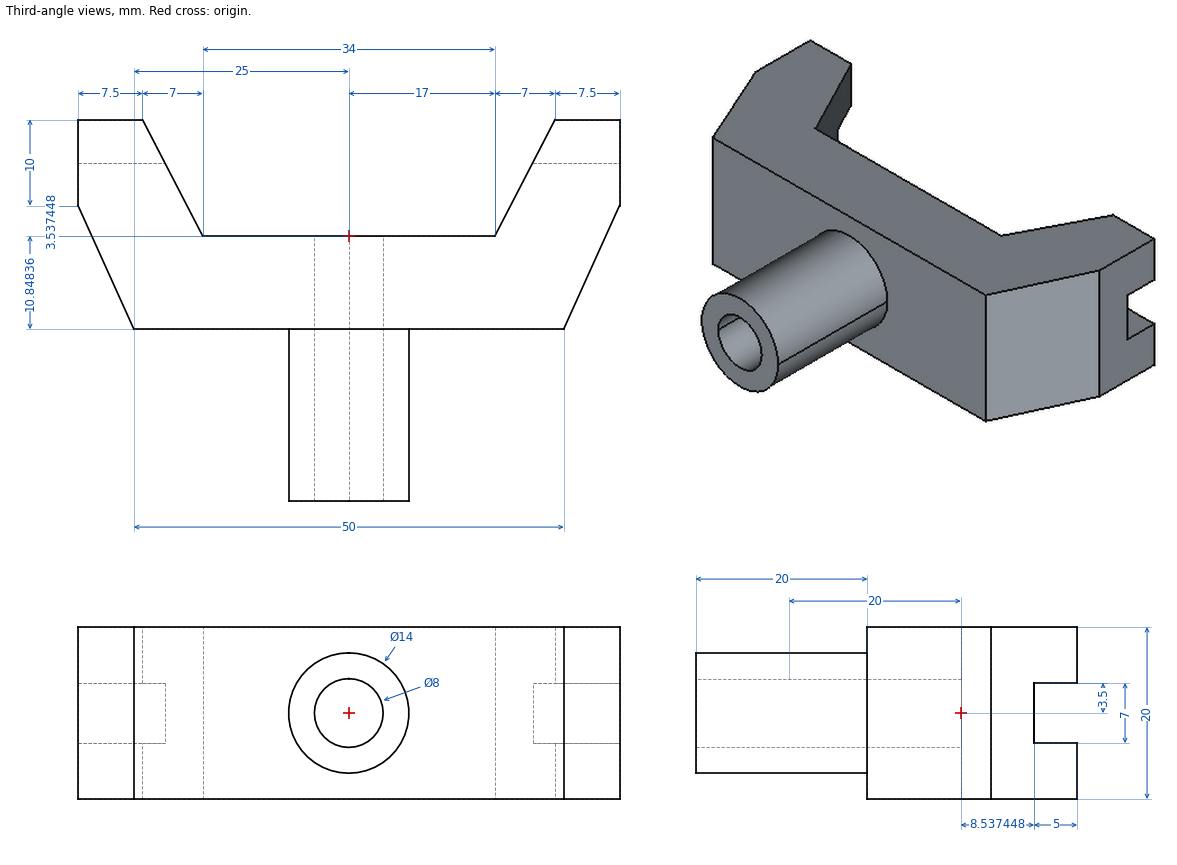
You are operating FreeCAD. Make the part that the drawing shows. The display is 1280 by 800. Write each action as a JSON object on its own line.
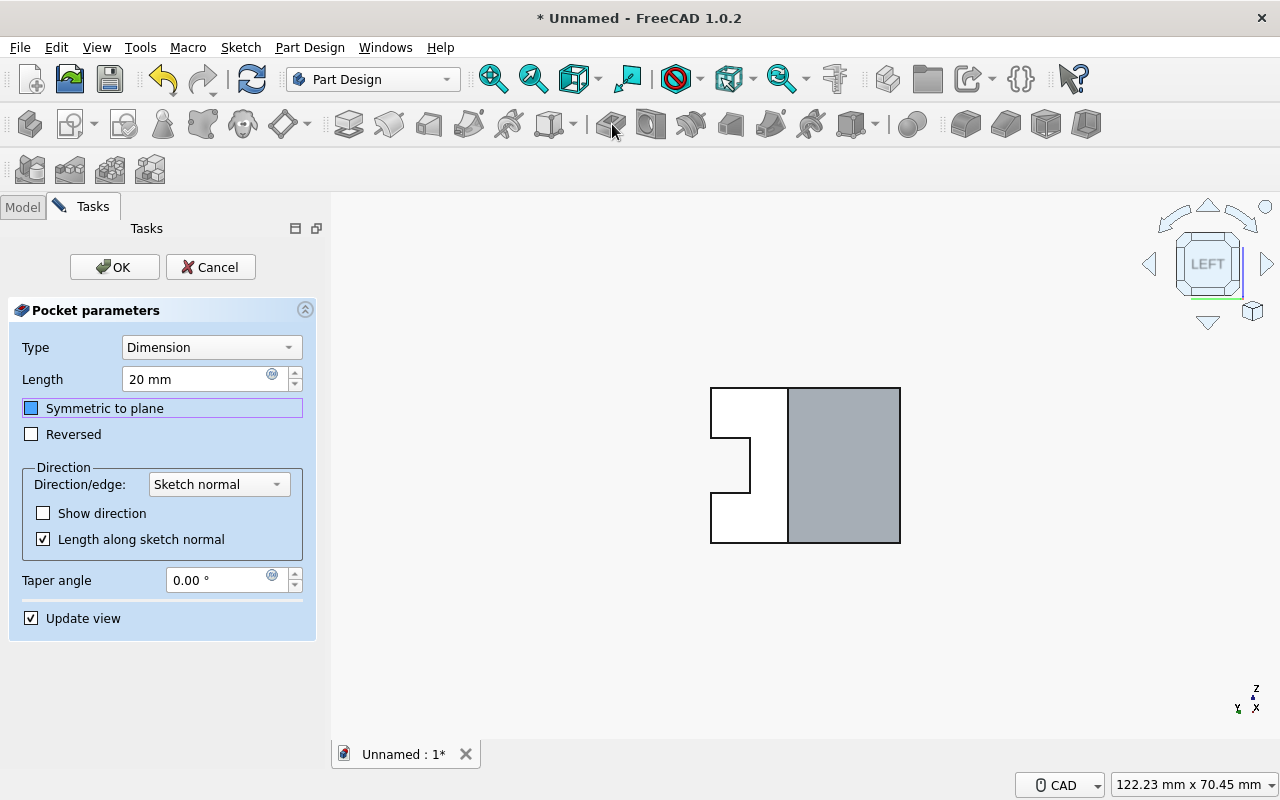
{"action": "left_click", "coordinate": [30, 434]}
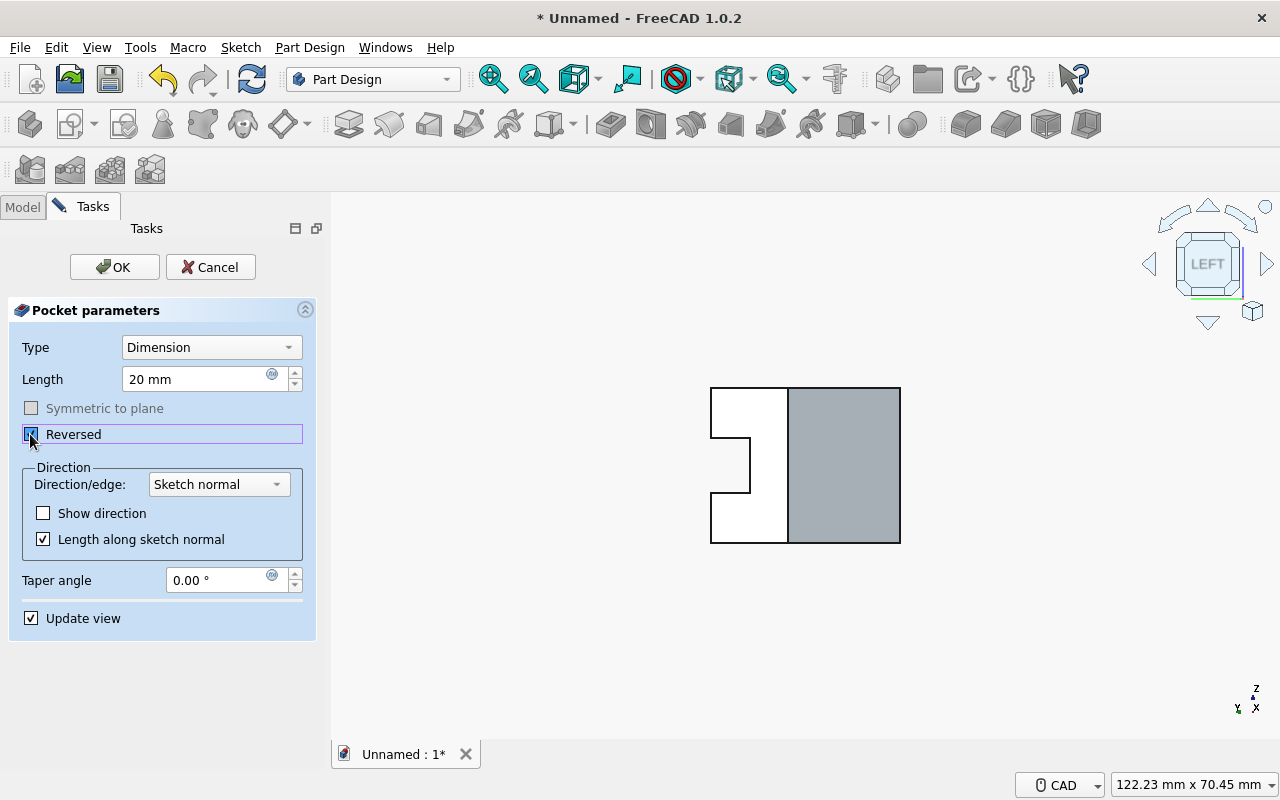
{"action": "left_click", "coordinate": [115, 267]}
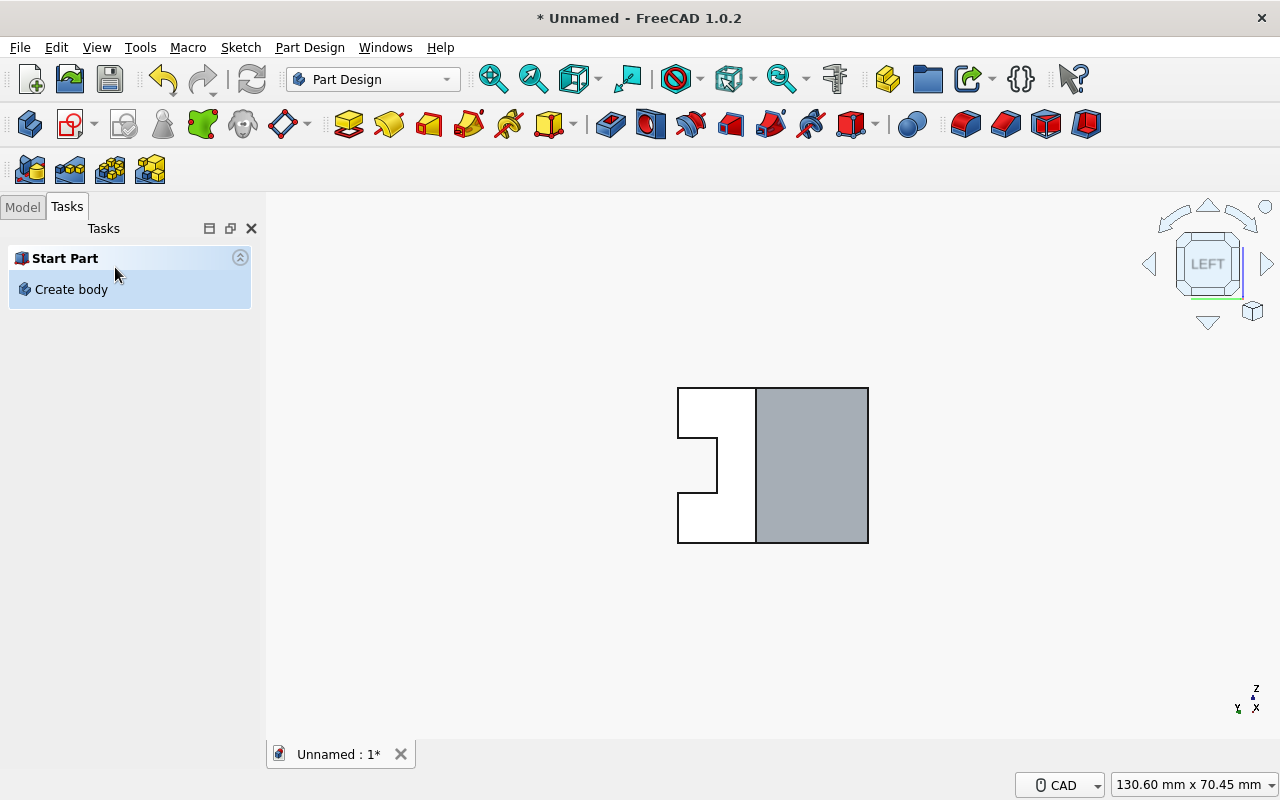
{"action": "left_click", "coordinate": [494, 80]}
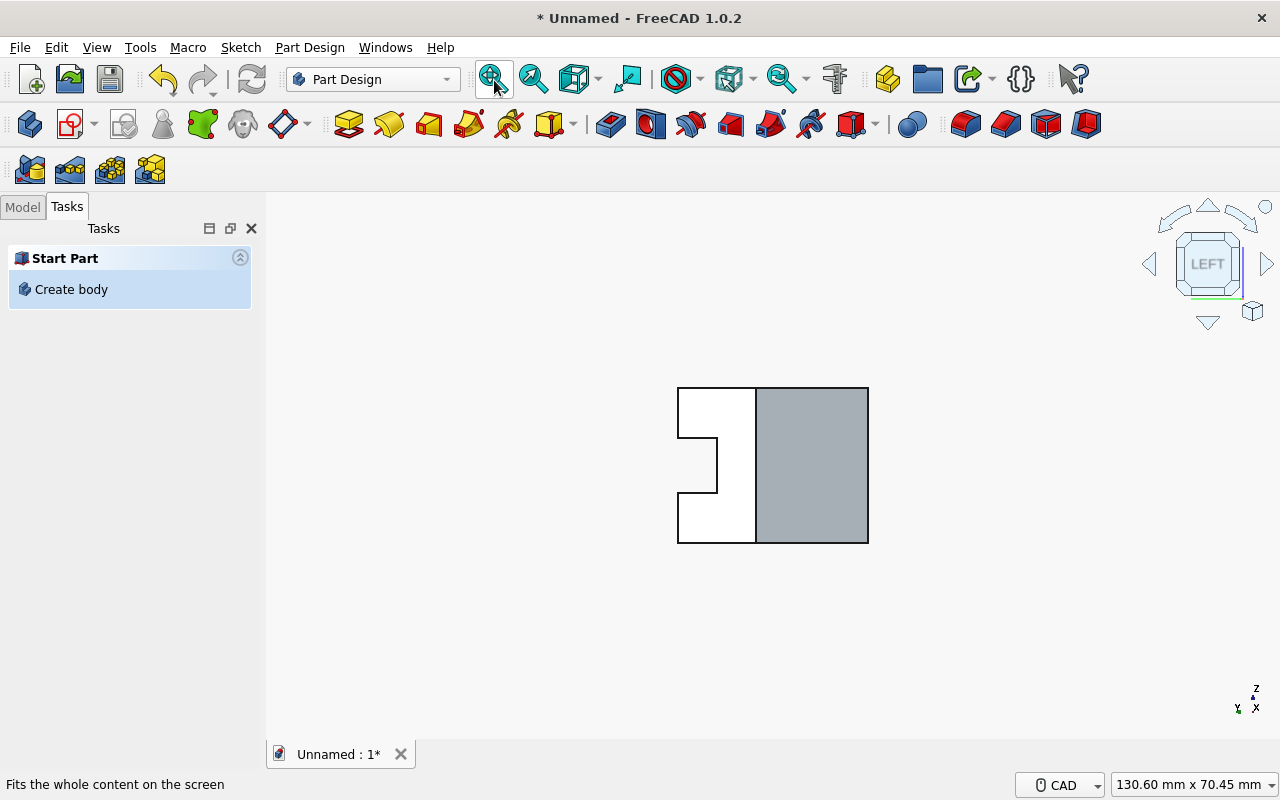
{"action": "key", "text": "0"}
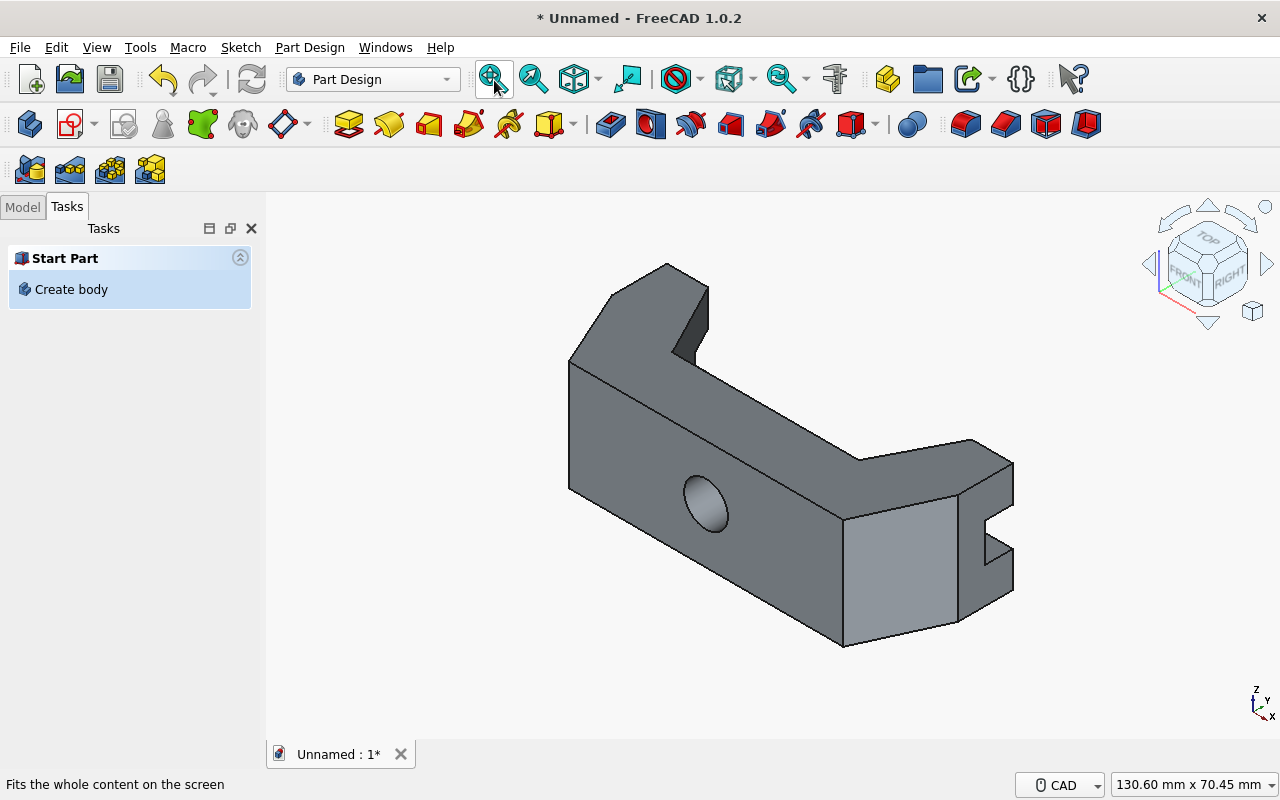
{"action": "left_click", "coordinate": [784, 548]}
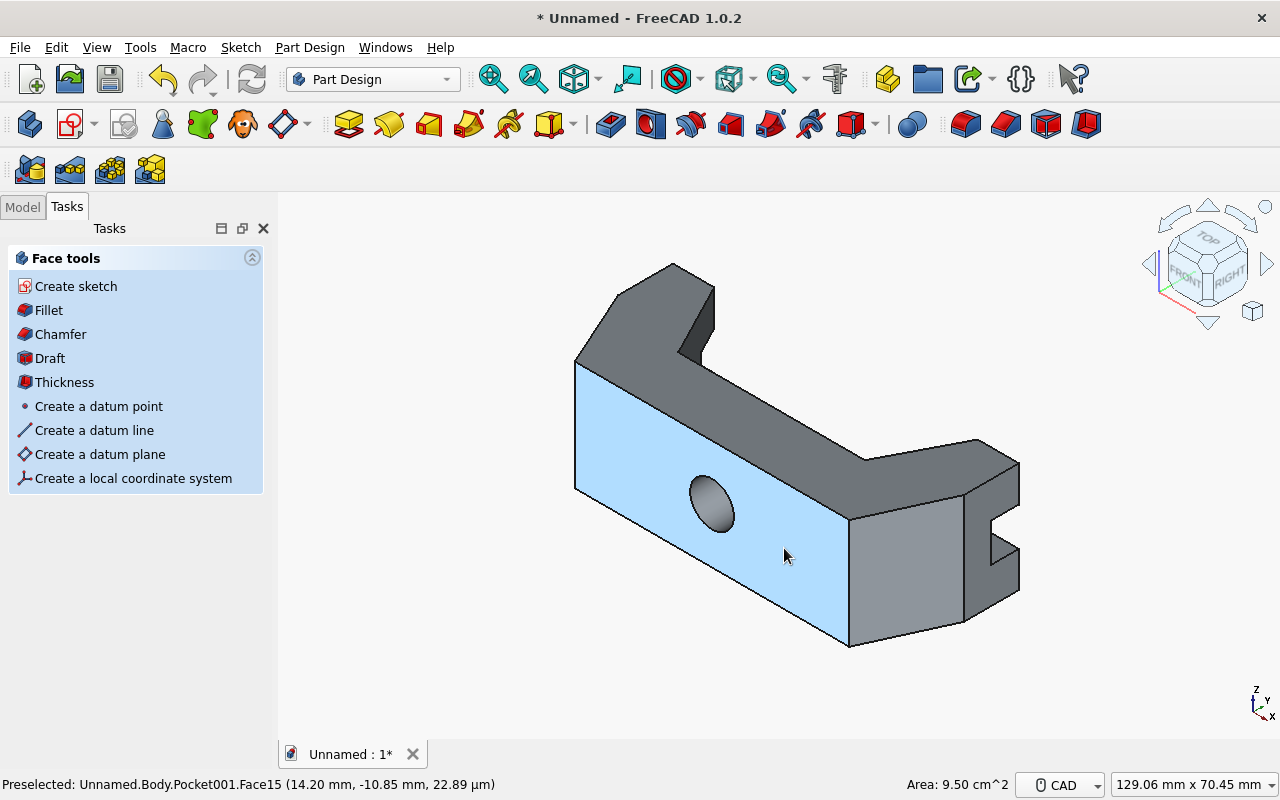
{"action": "left_click", "coordinate": [70, 124]}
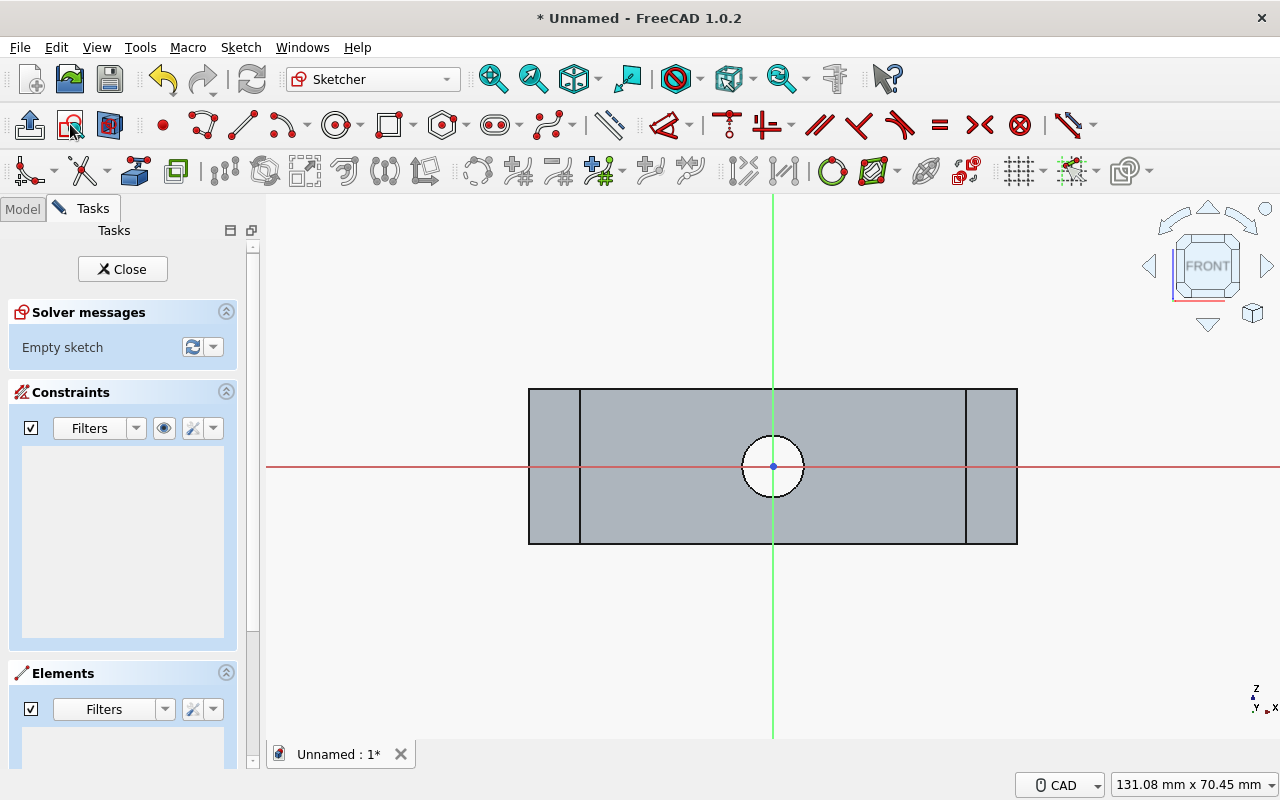
{"action": "scroll", "coordinate": [803, 467], "scroll_direction": "up", "scroll_amount": 6}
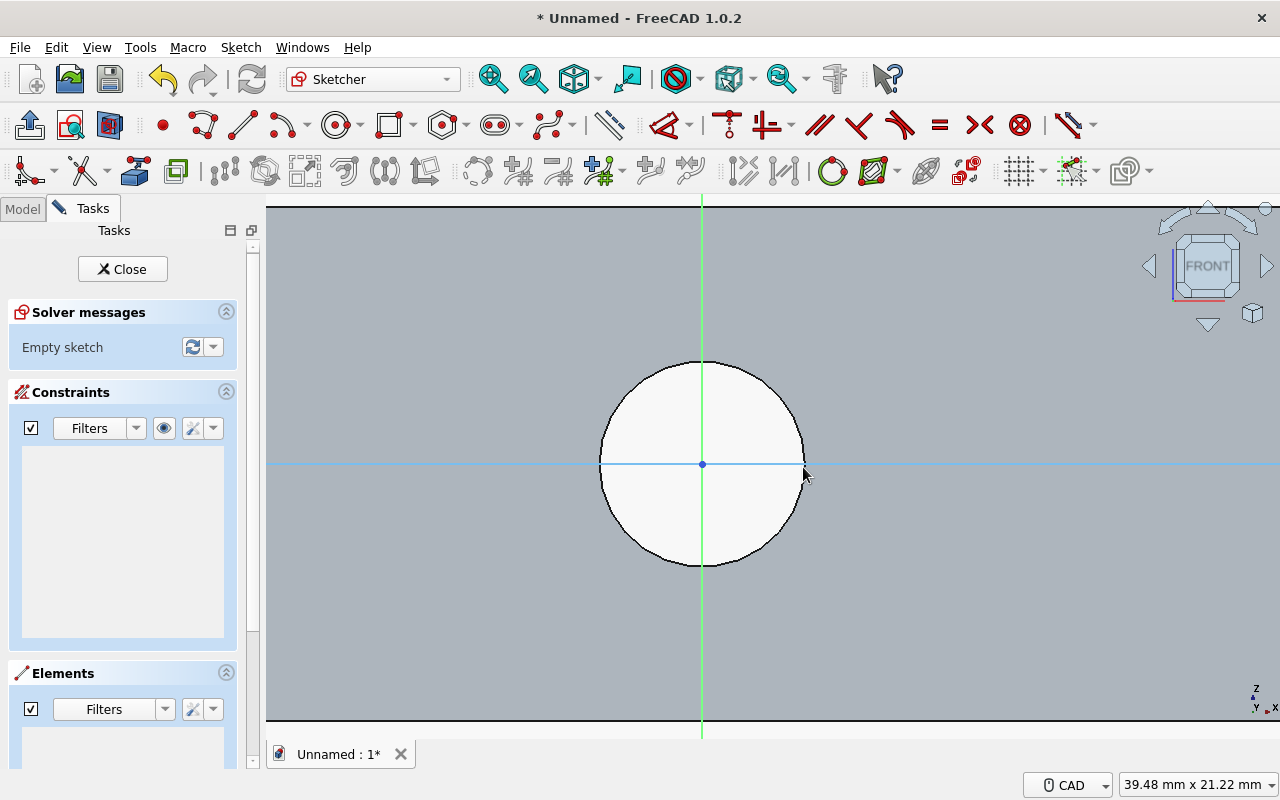
{"action": "left_click", "coordinate": [336, 126]}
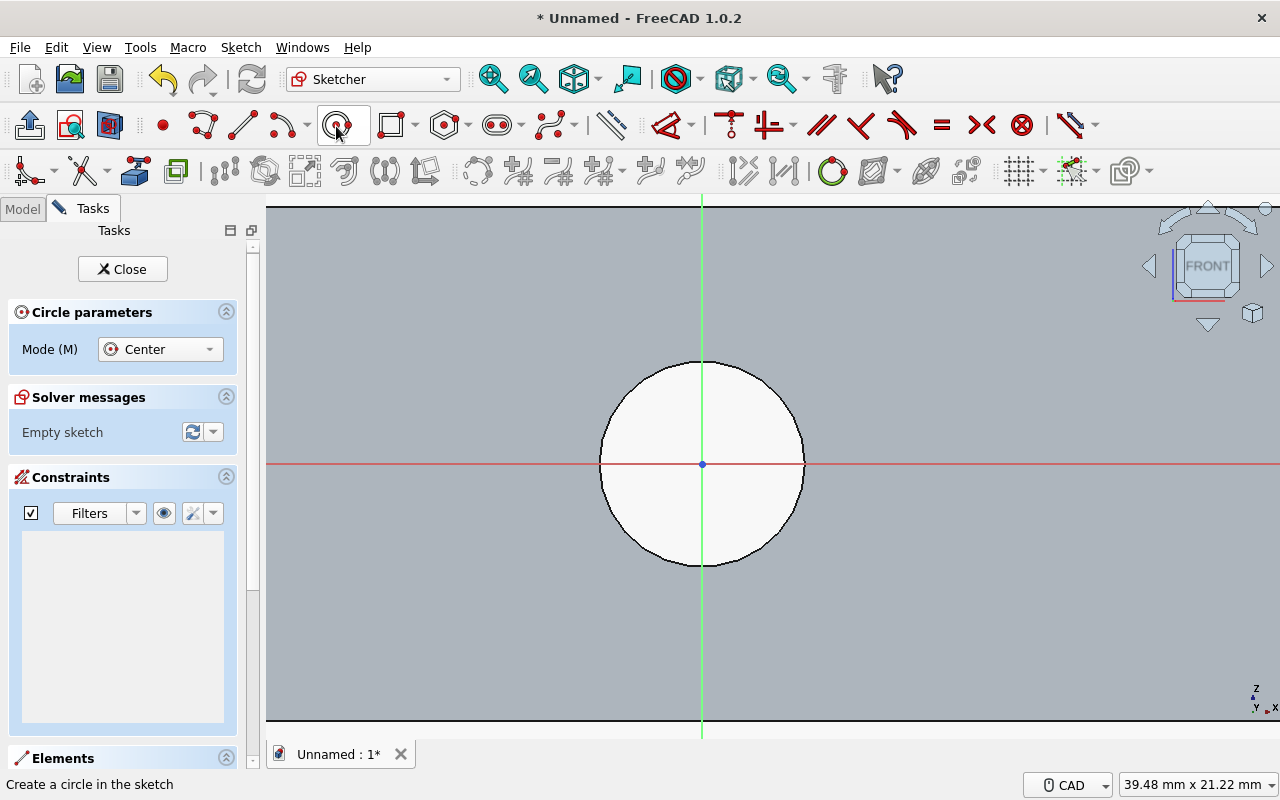
{"action": "left_click", "coordinate": [702, 464]}
{"action": "mouse_move", "coordinate": [829, 337]}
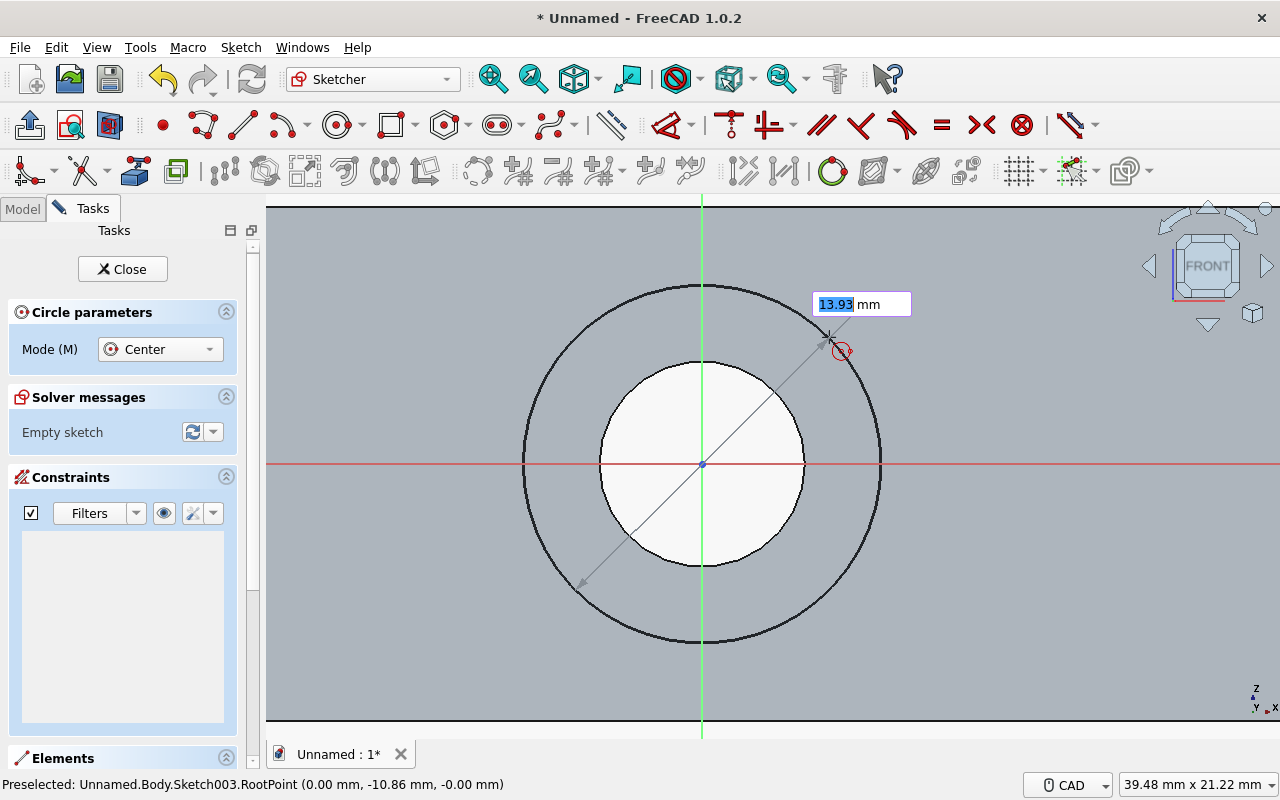
{"action": "type", "text": "14"}
{"action": "key", "text": "Return"}
{"action": "key", "text": "Escape"}